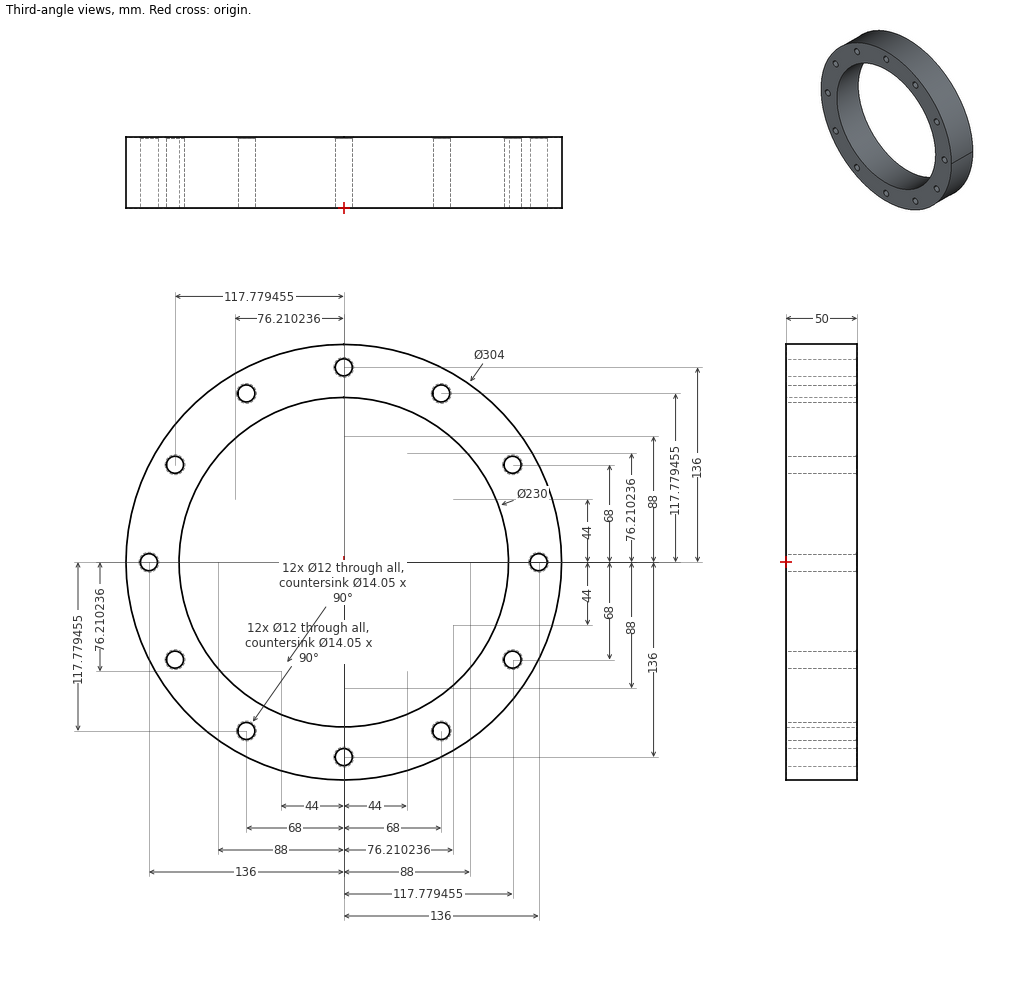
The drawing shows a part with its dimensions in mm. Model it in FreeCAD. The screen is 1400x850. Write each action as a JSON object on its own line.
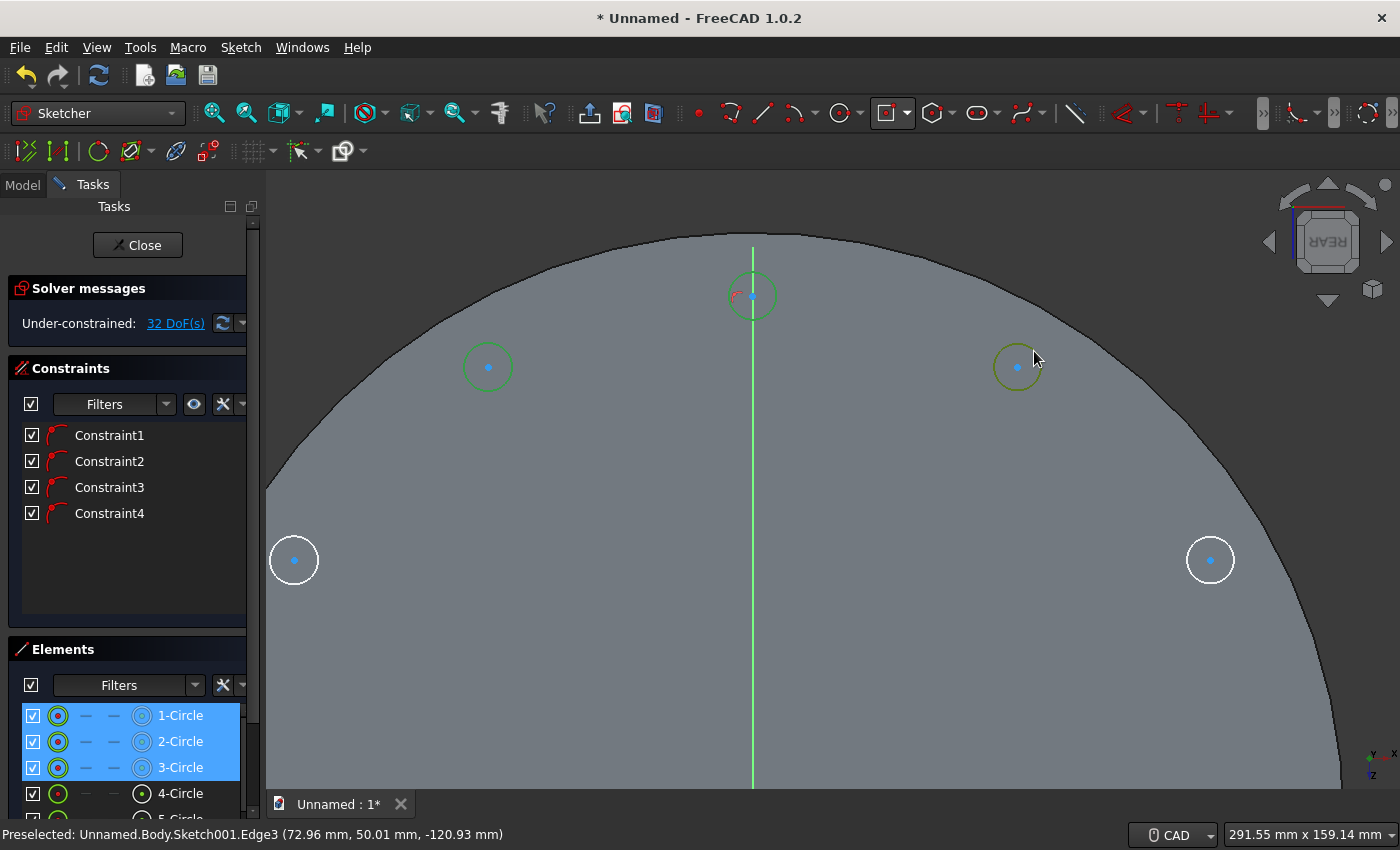
{"action": "left_click", "coordinate": [1227, 544]}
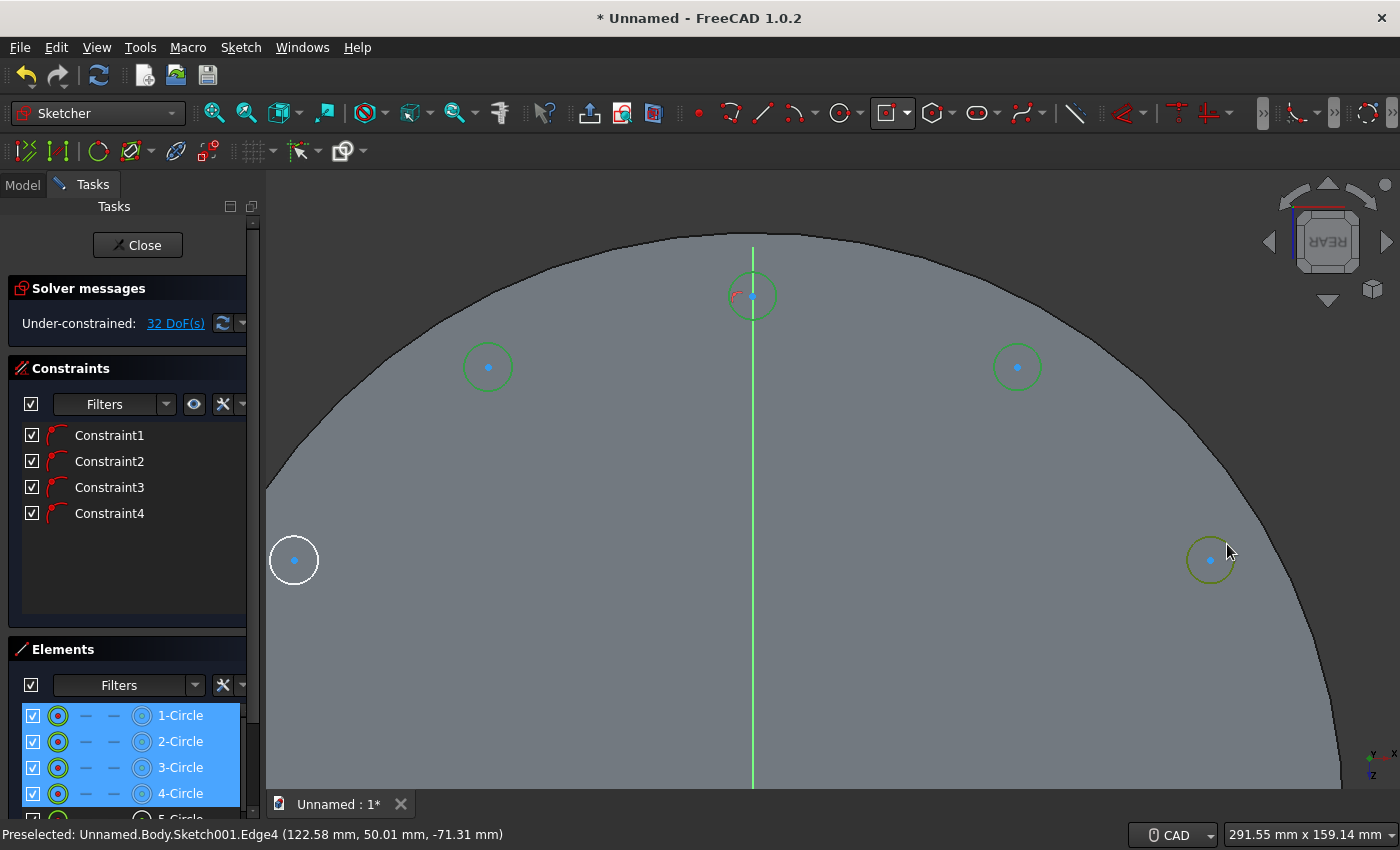
{"action": "scroll", "coordinate": [771, 279], "scroll_direction": "down", "scroll_amount": 5}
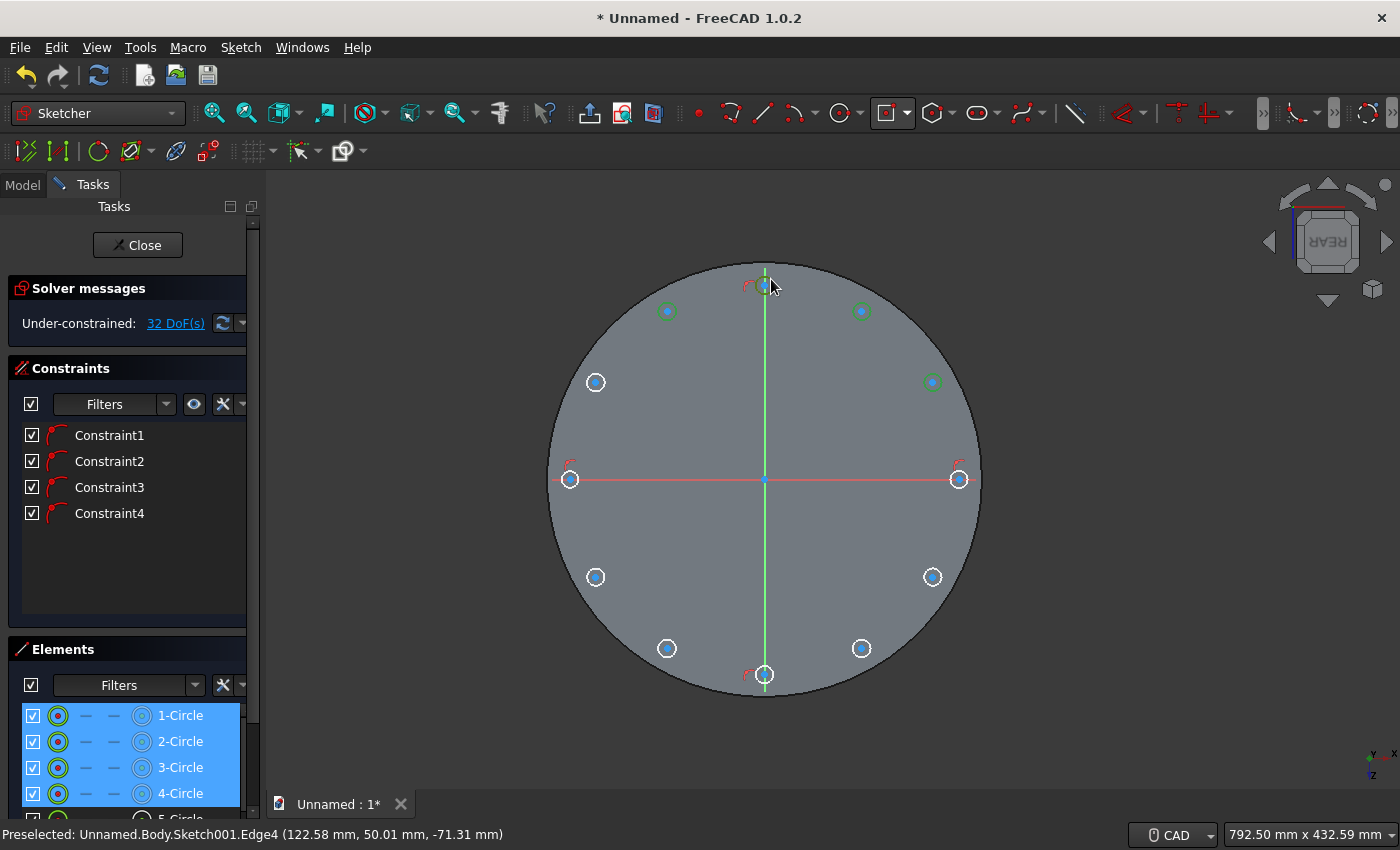
{"action": "scroll", "coordinate": [965, 473], "scroll_direction": "up", "scroll_amount": 5}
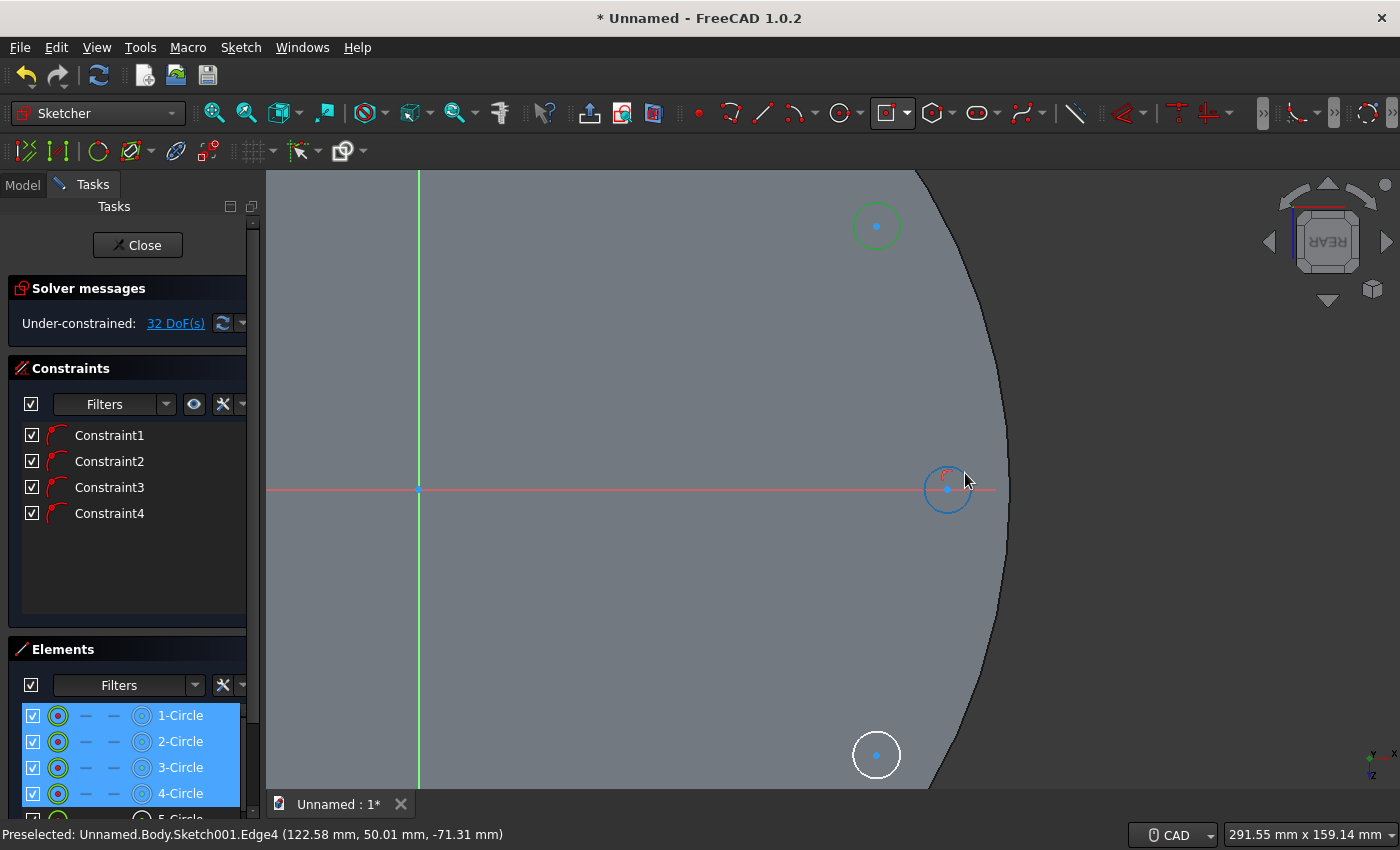
{"action": "left_click", "coordinate": [964, 473]}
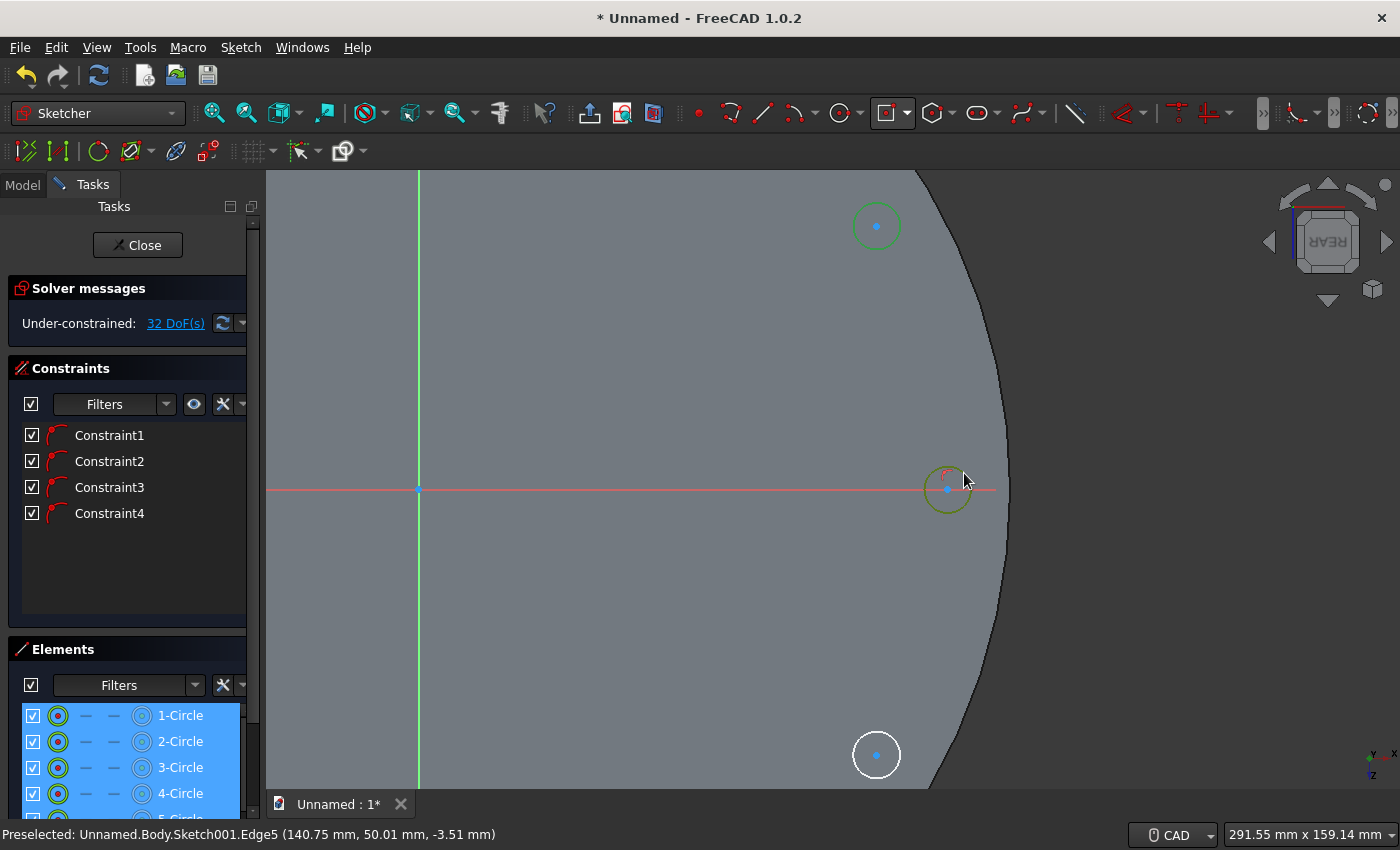
{"action": "left_click", "coordinate": [893, 738]}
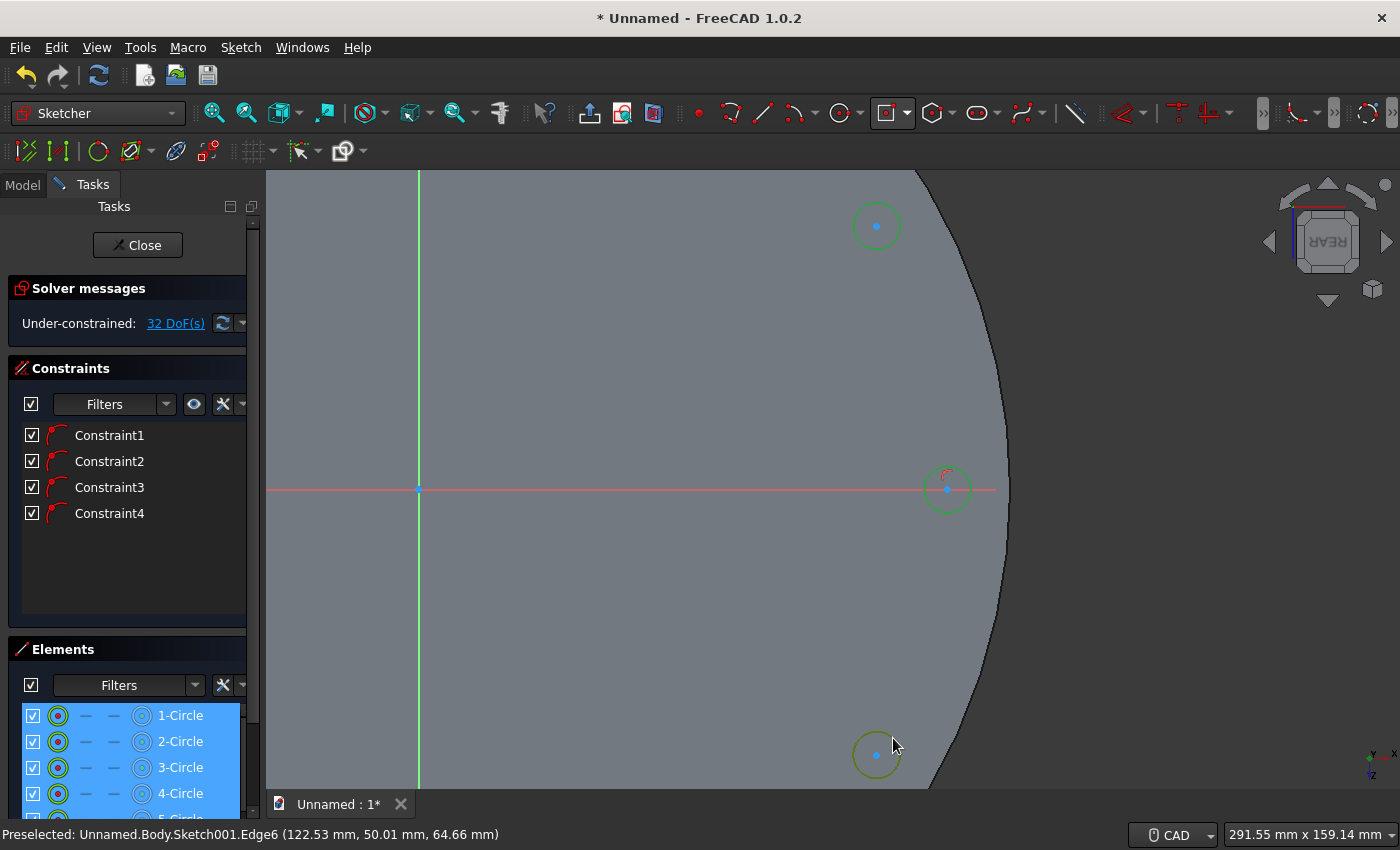
{"action": "scroll", "coordinate": [966, 473], "scroll_direction": "down", "scroll_amount": 5}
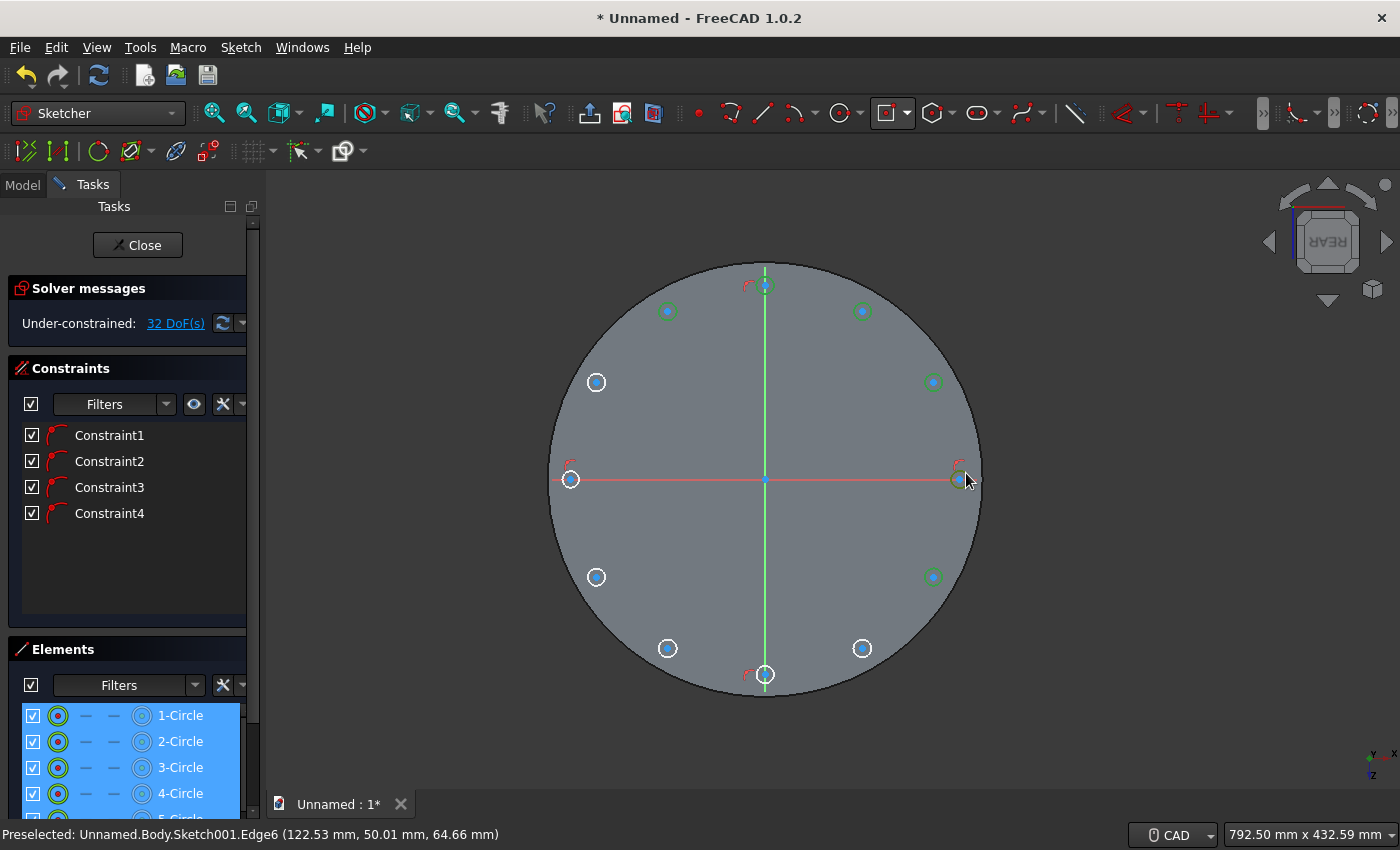
{"action": "scroll", "coordinate": [869, 642], "scroll_direction": "up", "scroll_amount": 3}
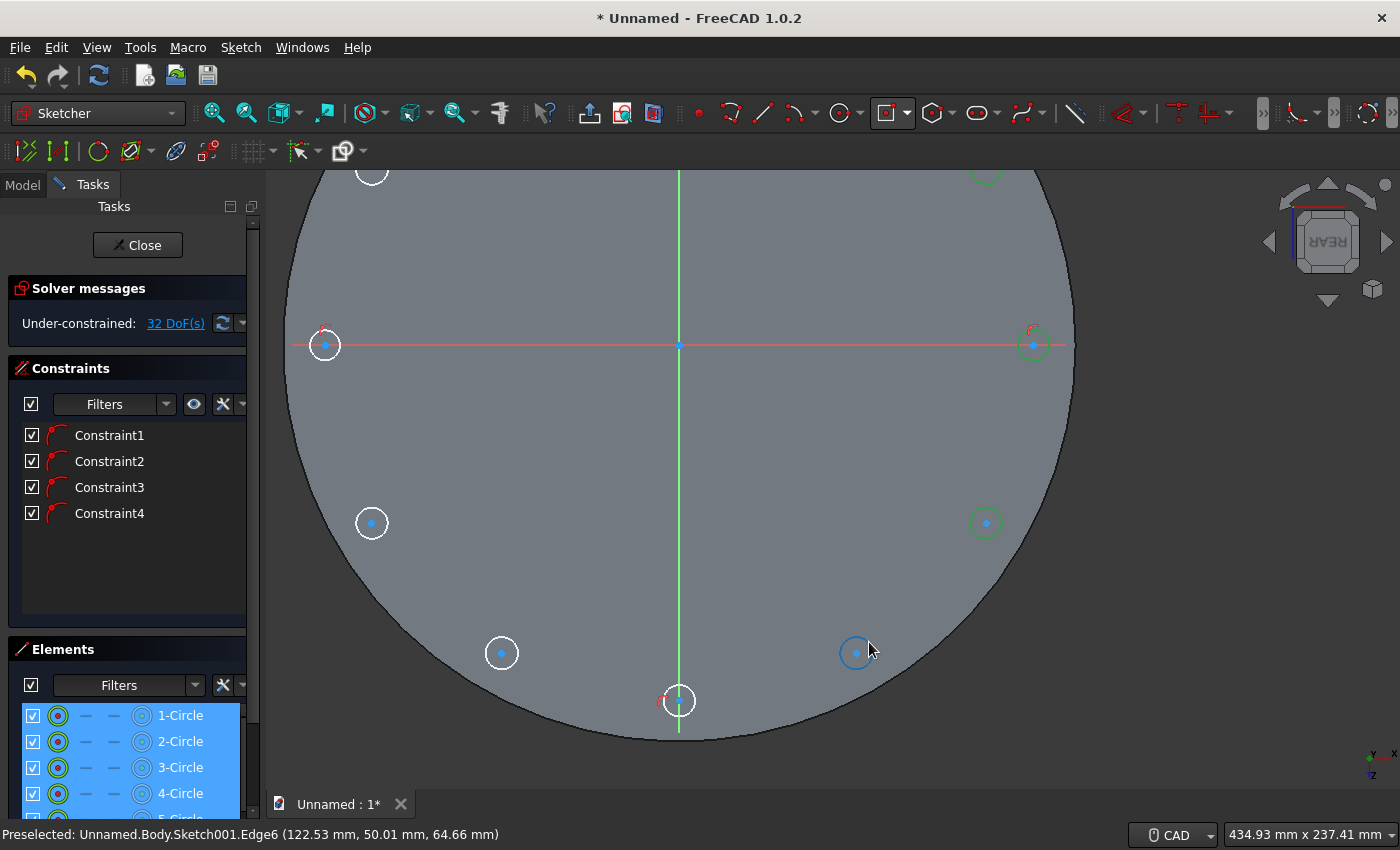
{"action": "left_click", "coordinate": [868, 642]}